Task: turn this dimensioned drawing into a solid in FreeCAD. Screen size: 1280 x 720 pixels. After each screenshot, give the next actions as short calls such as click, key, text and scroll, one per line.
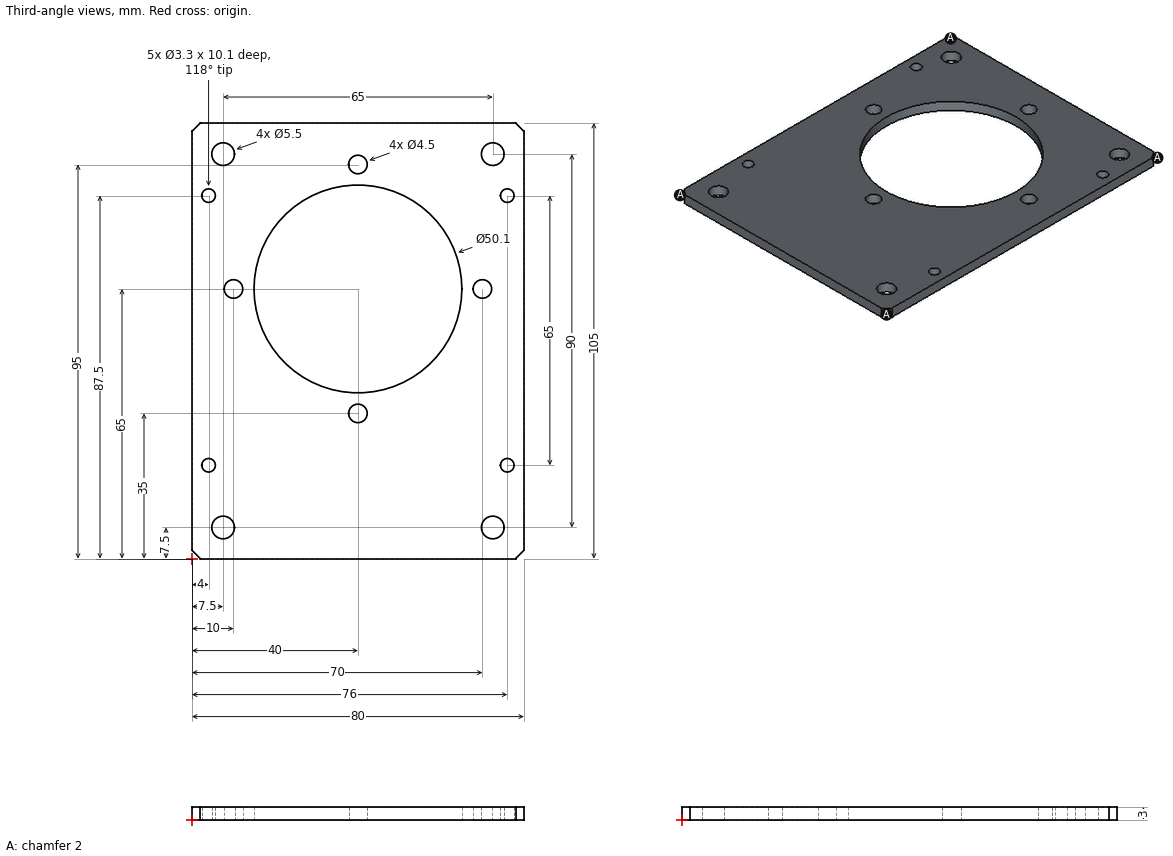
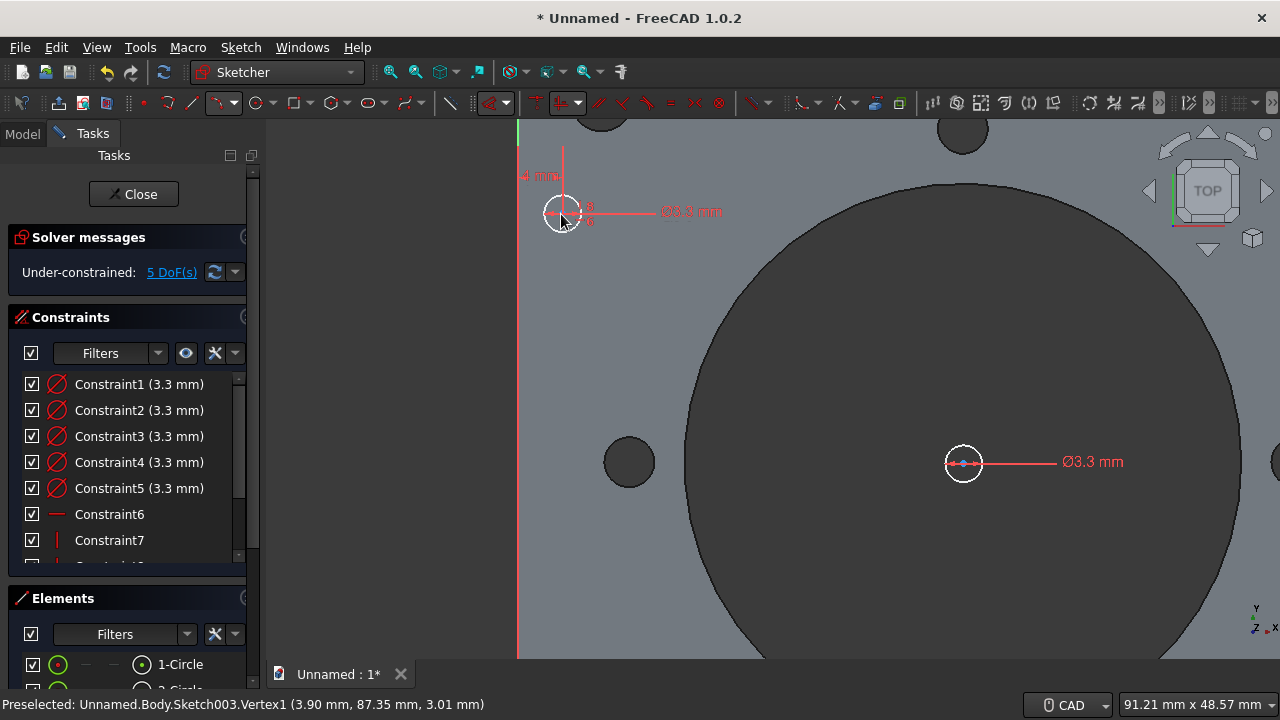
scroll(562, 214, down, 5)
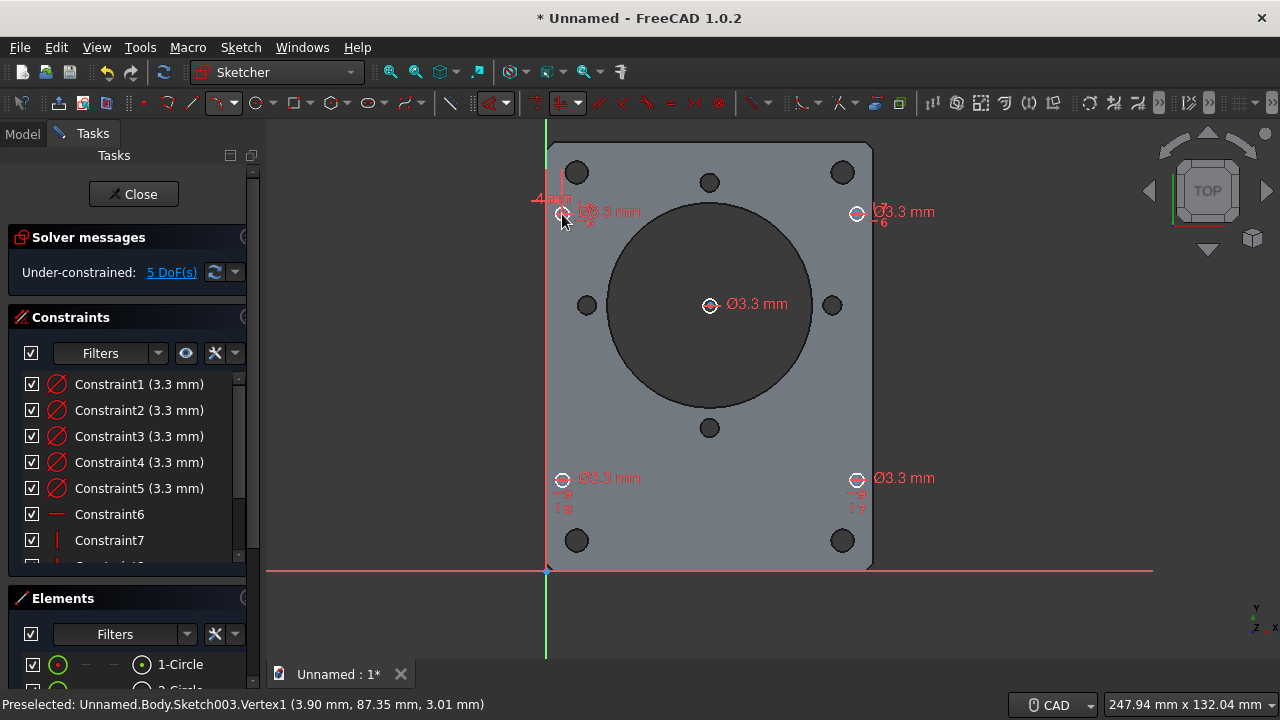
click(857, 214)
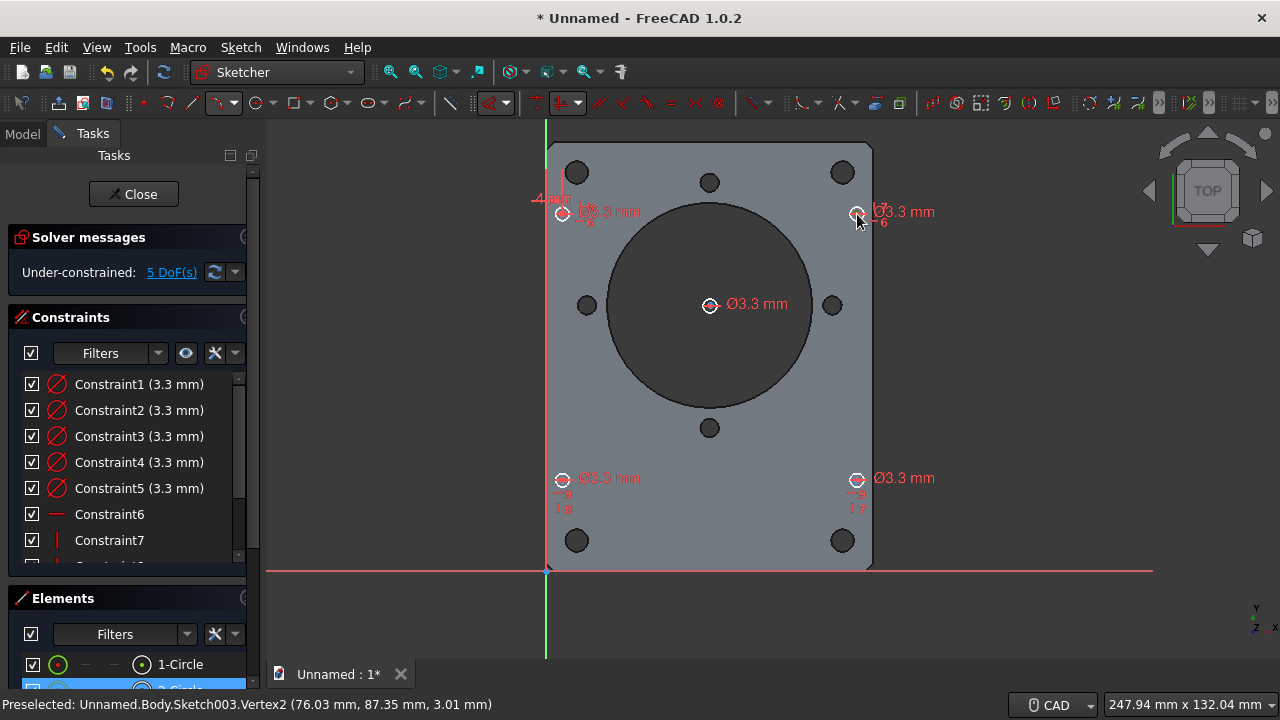
click(508, 104)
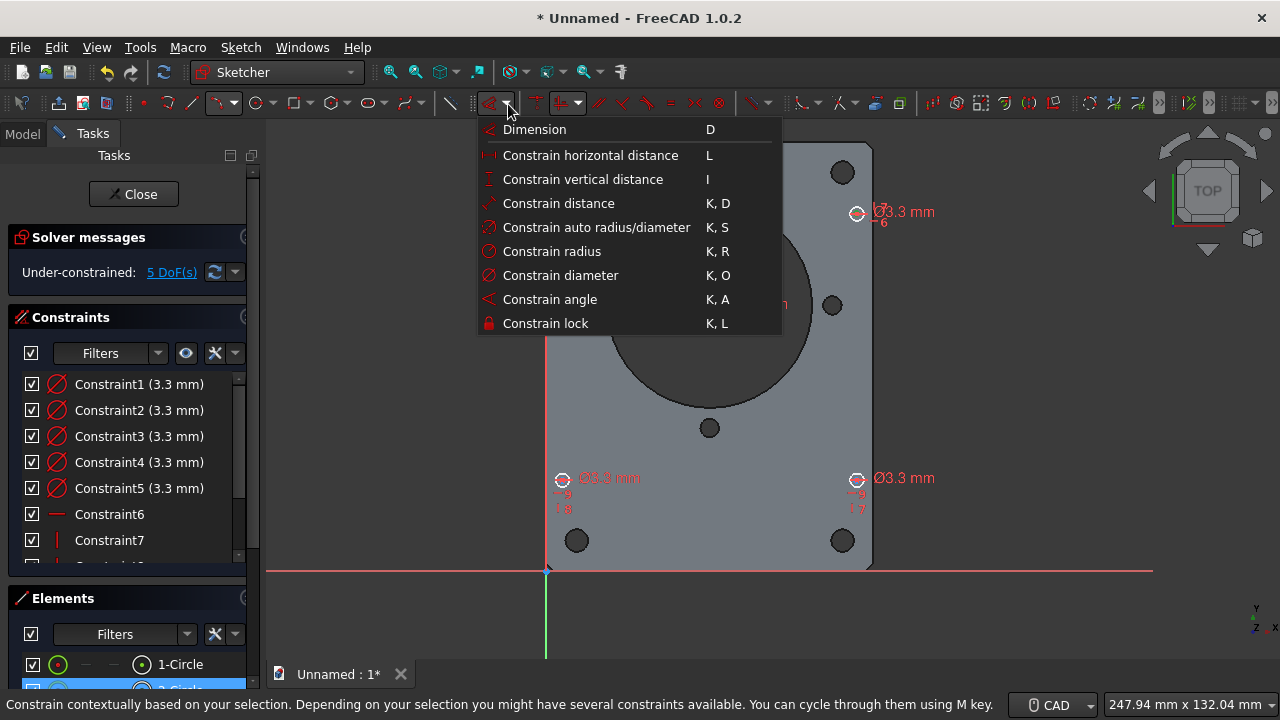
click(630, 155)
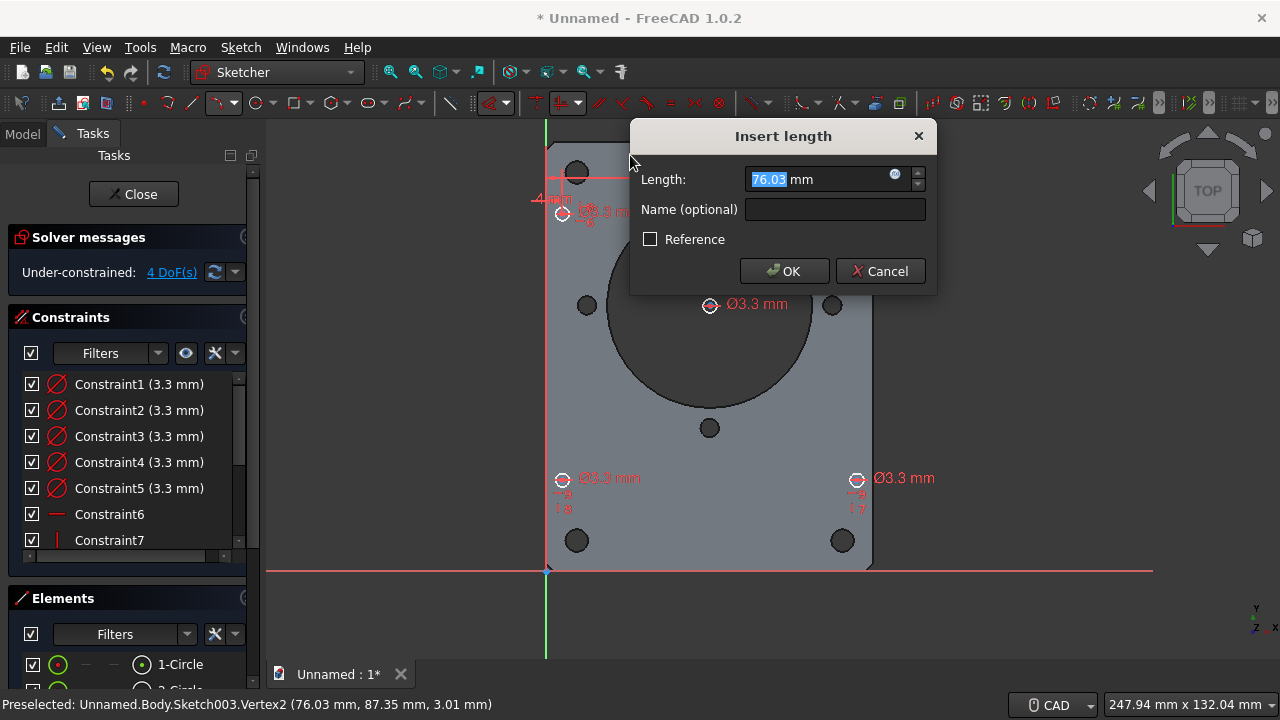
text(76)
key(Return)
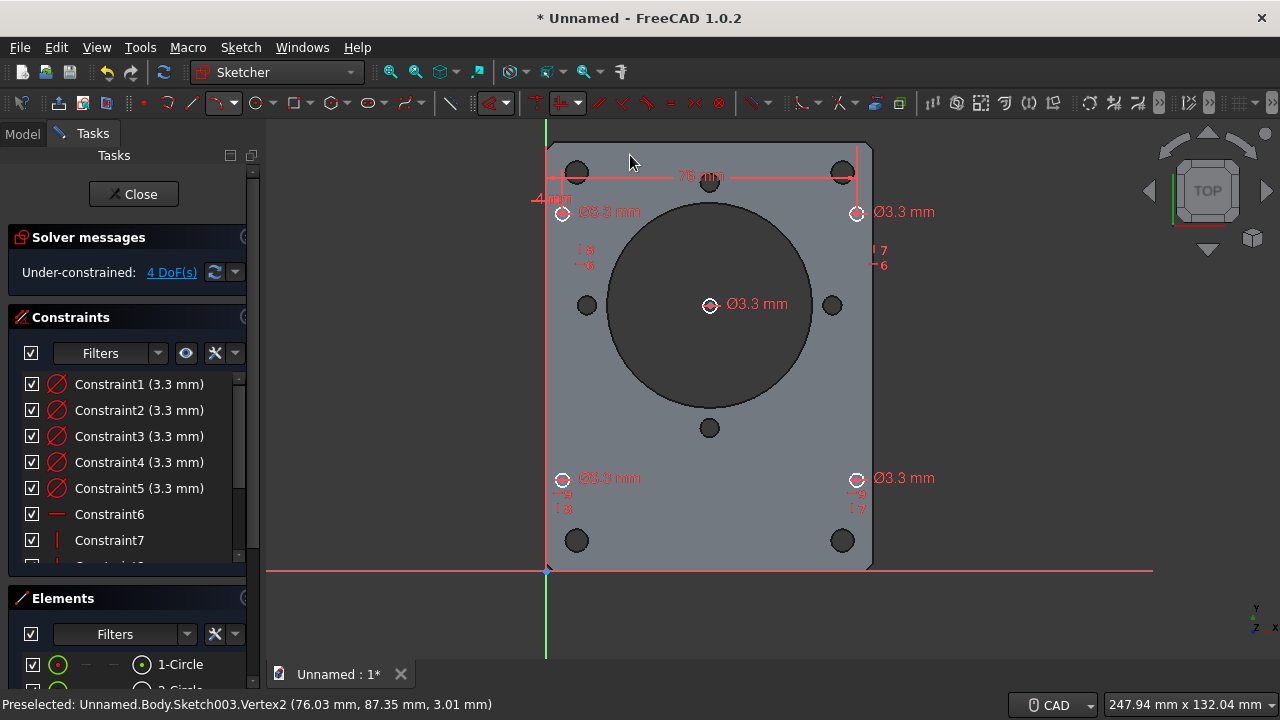
click(710, 306)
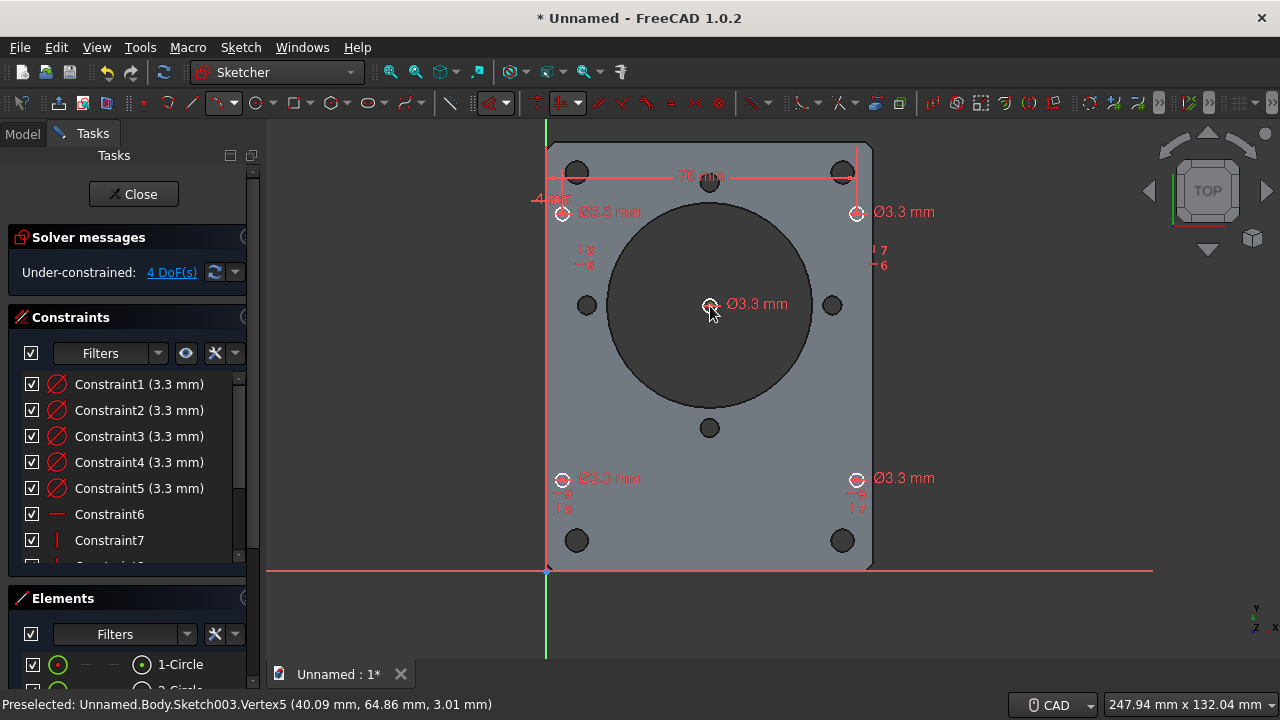
key(l)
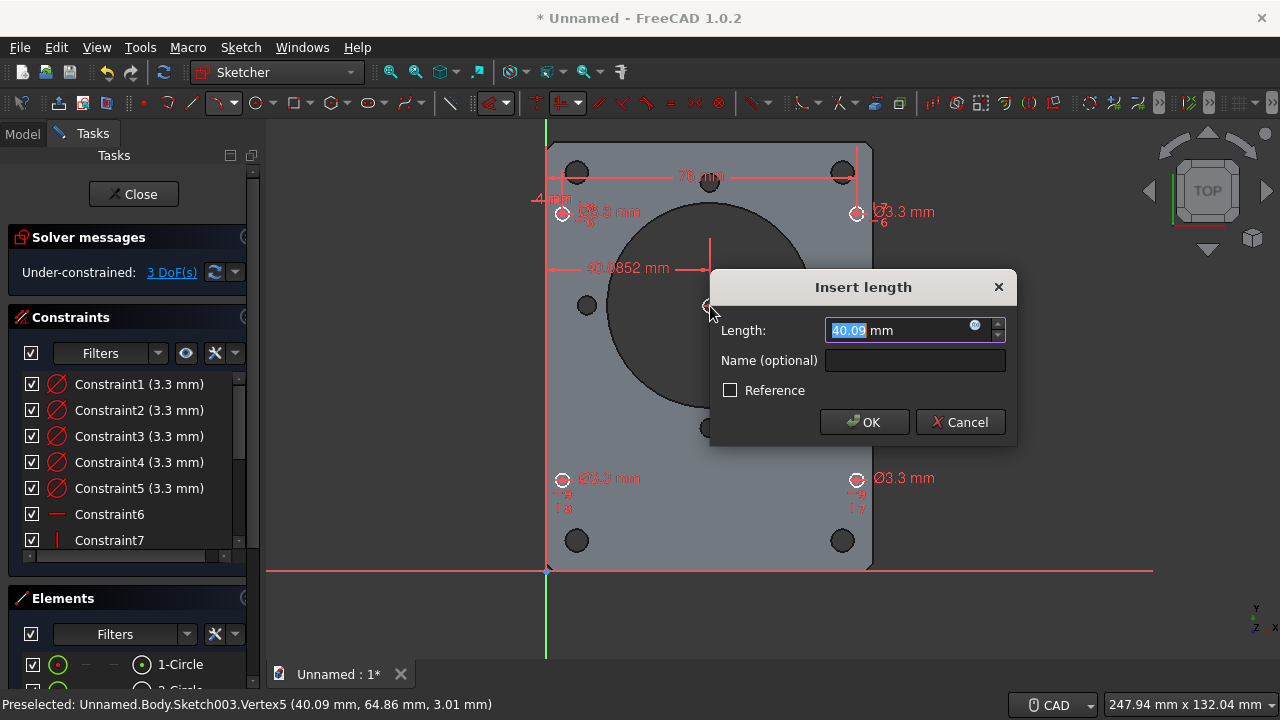
text(40)
key(Return)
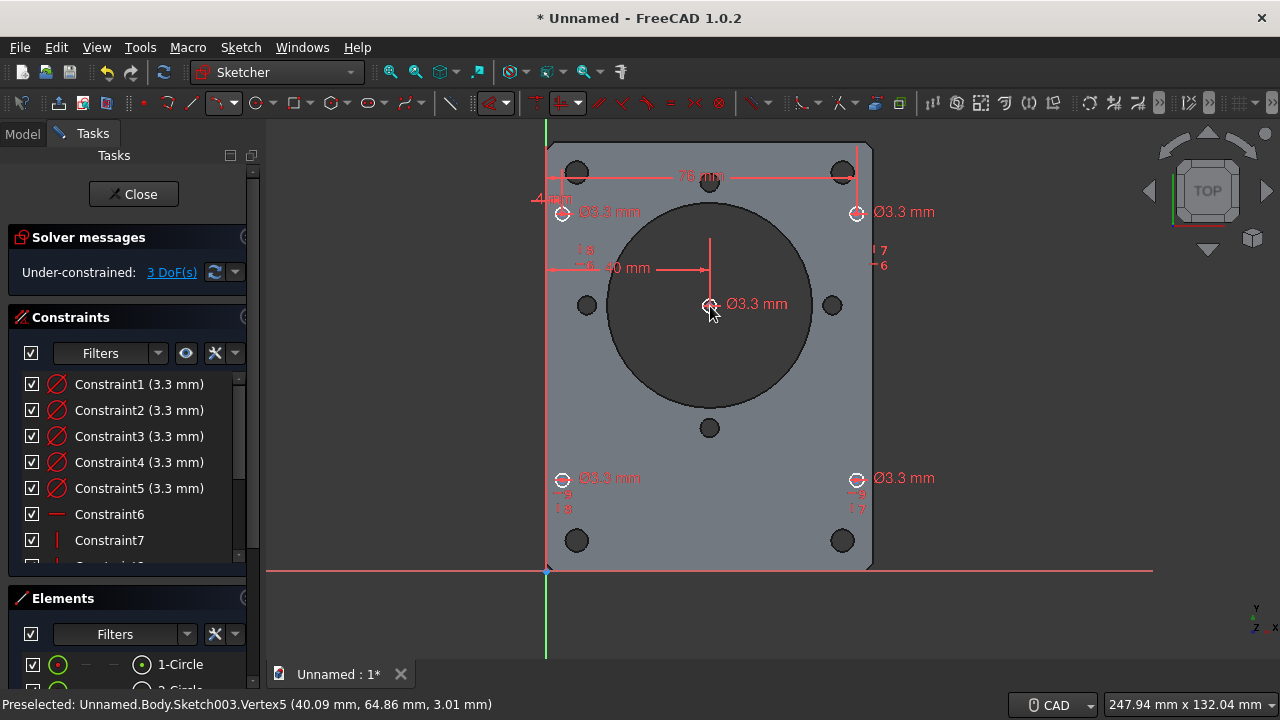
click(710, 306)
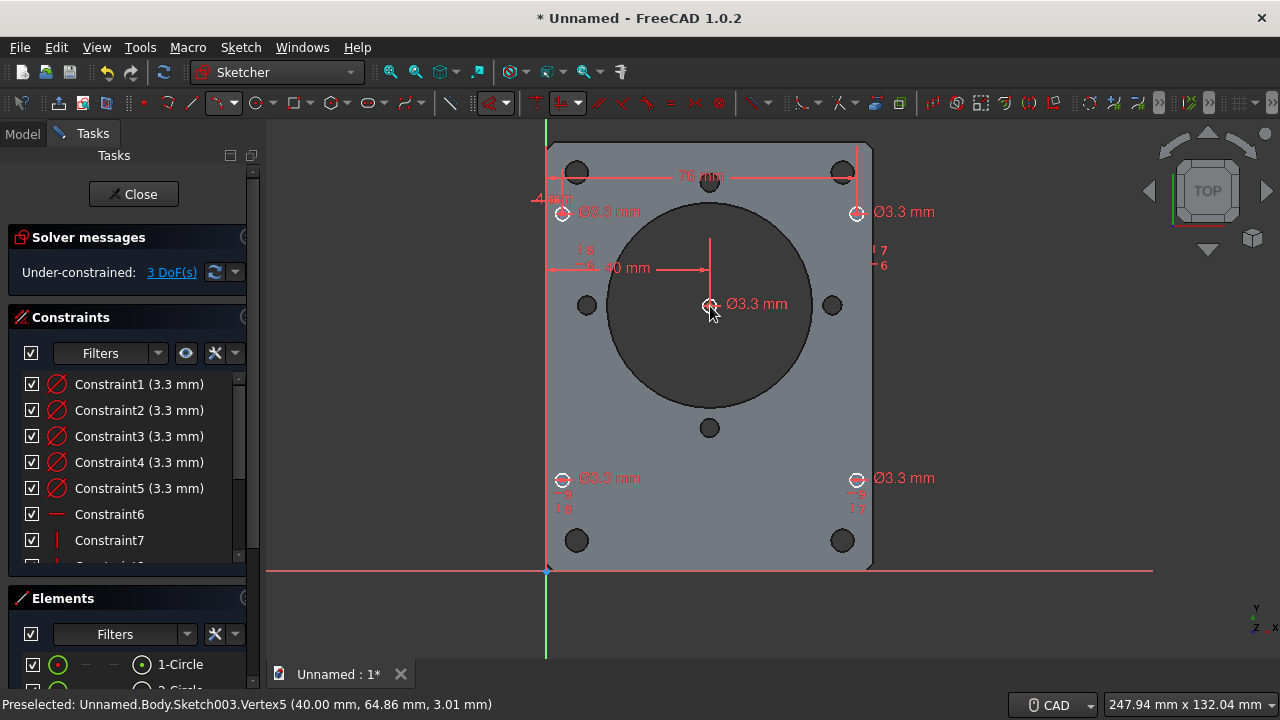
key(i)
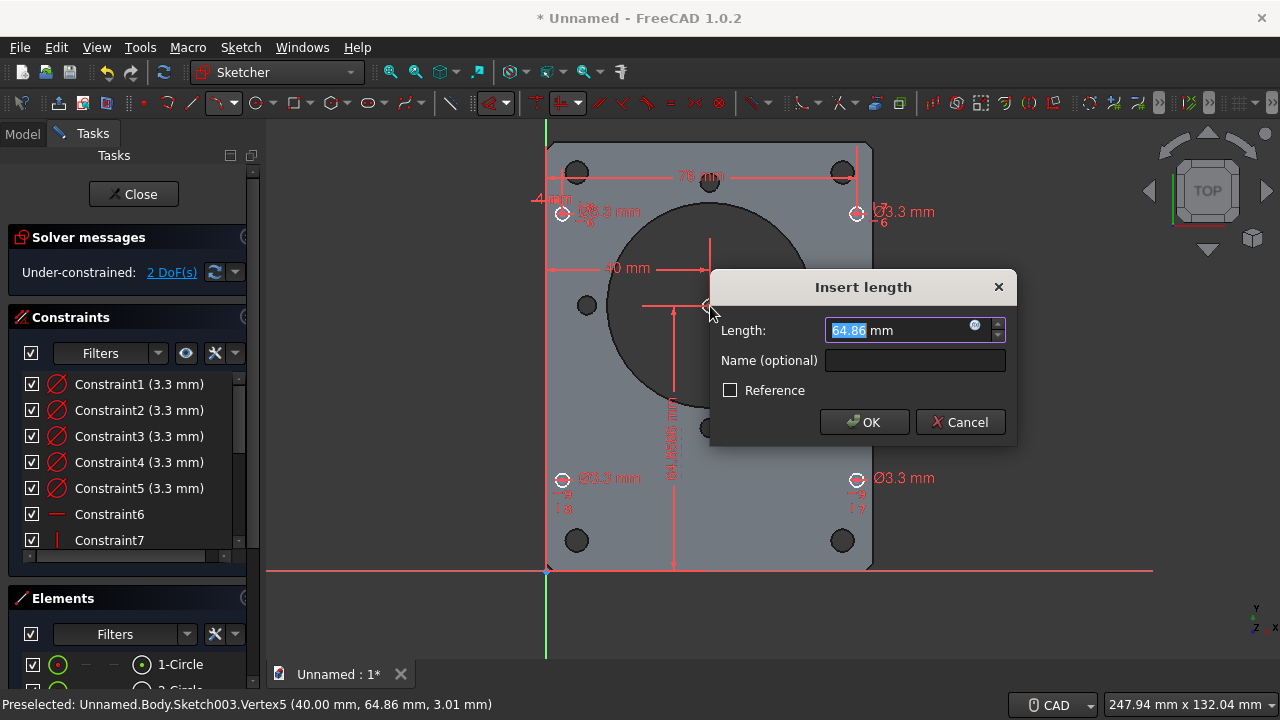
text(65)
key(Return)